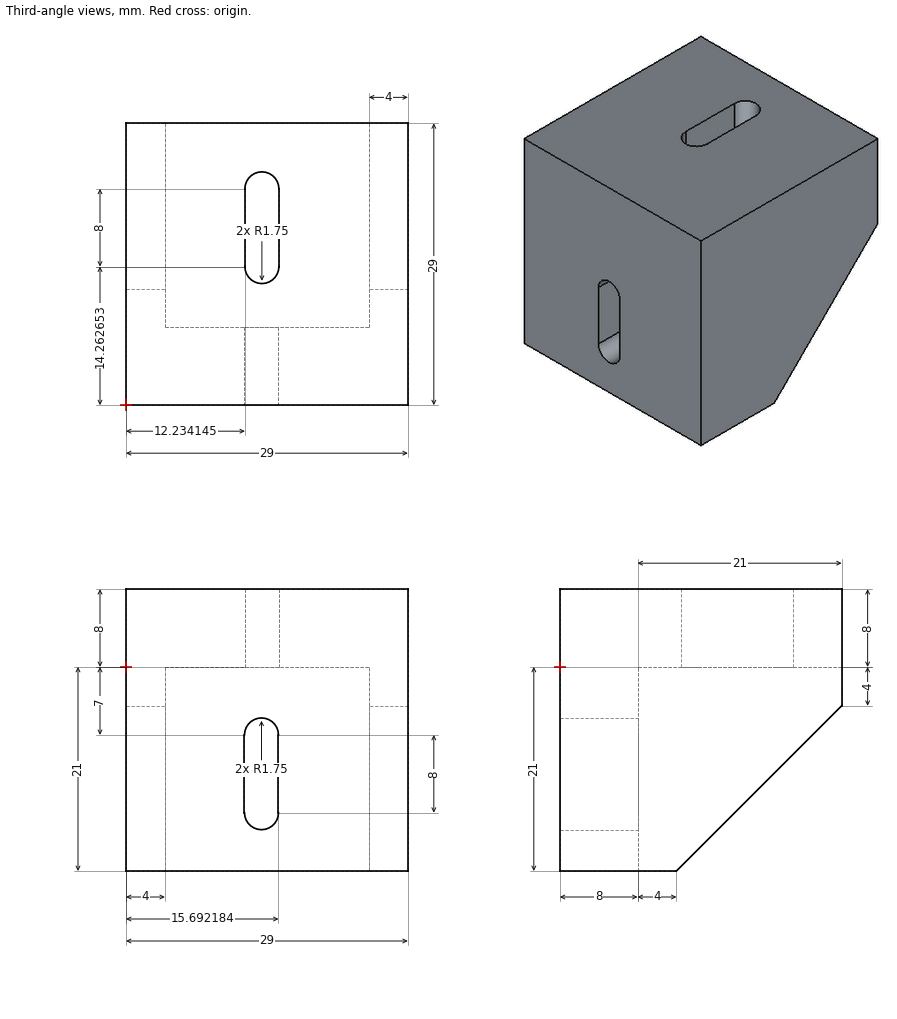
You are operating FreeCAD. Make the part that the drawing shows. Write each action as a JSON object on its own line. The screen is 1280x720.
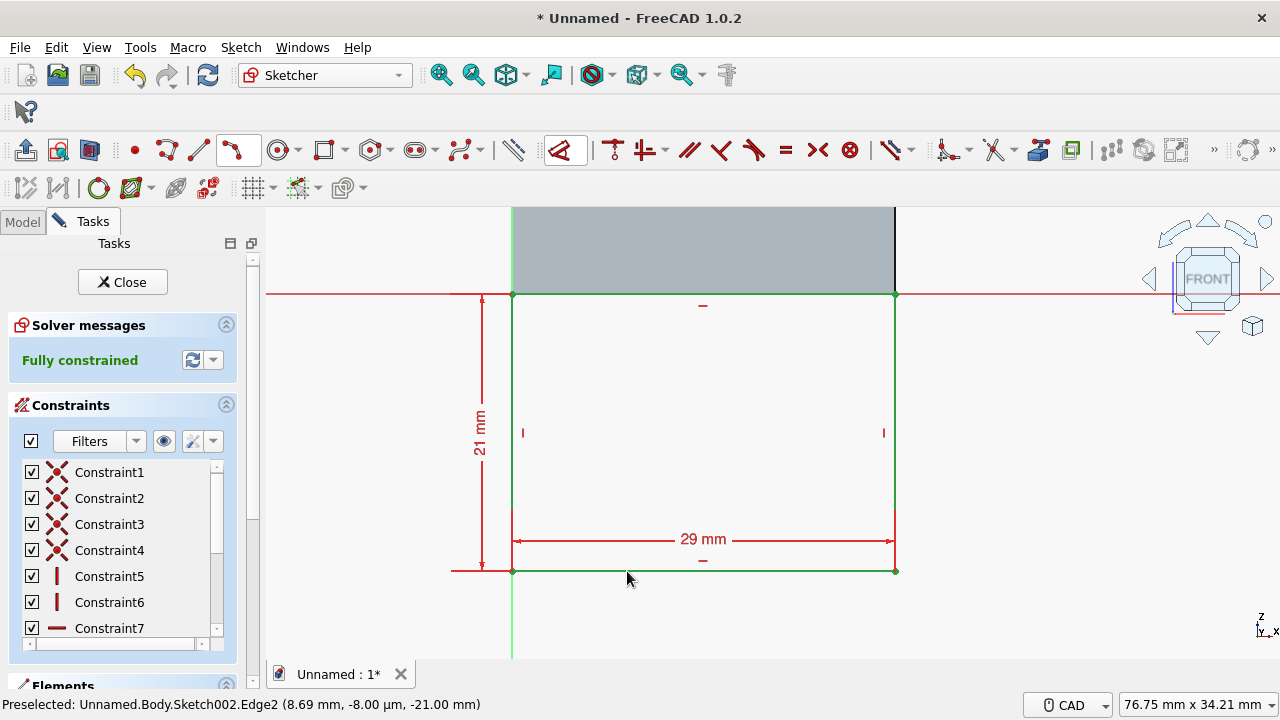
{"action": "left_click", "coordinate": [123, 282]}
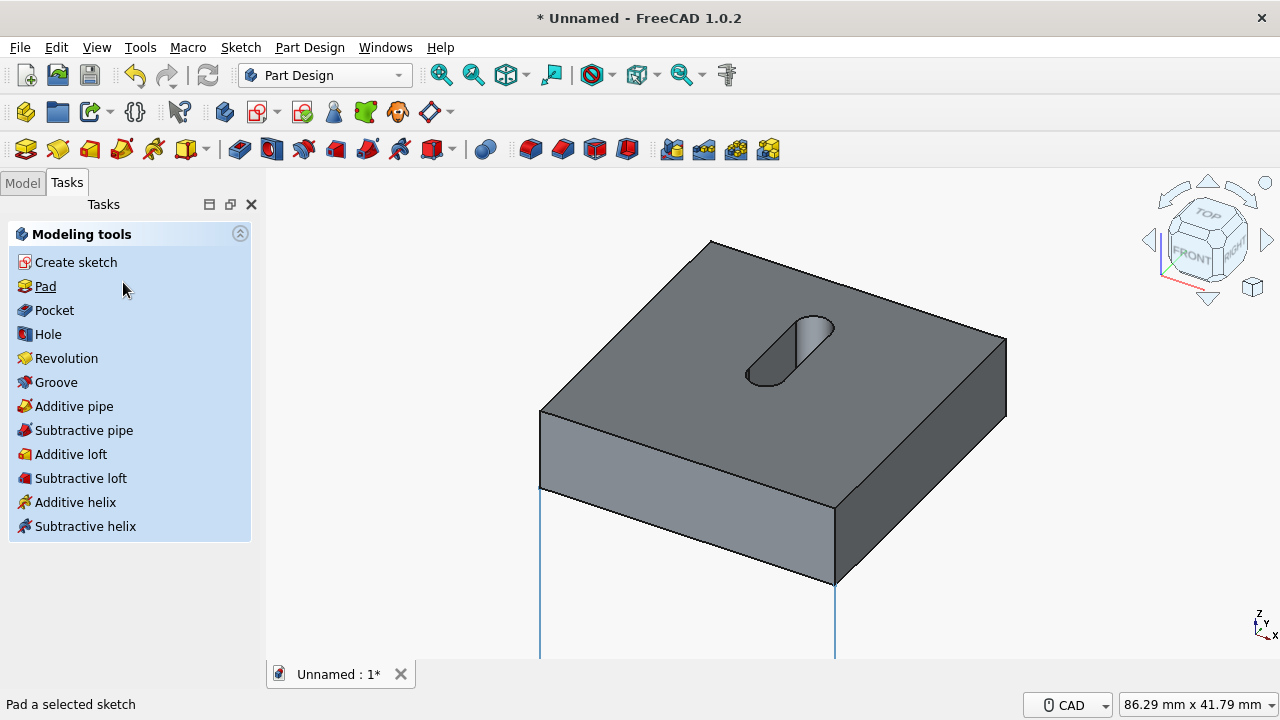
{"action": "left_click", "coordinate": [26, 150]}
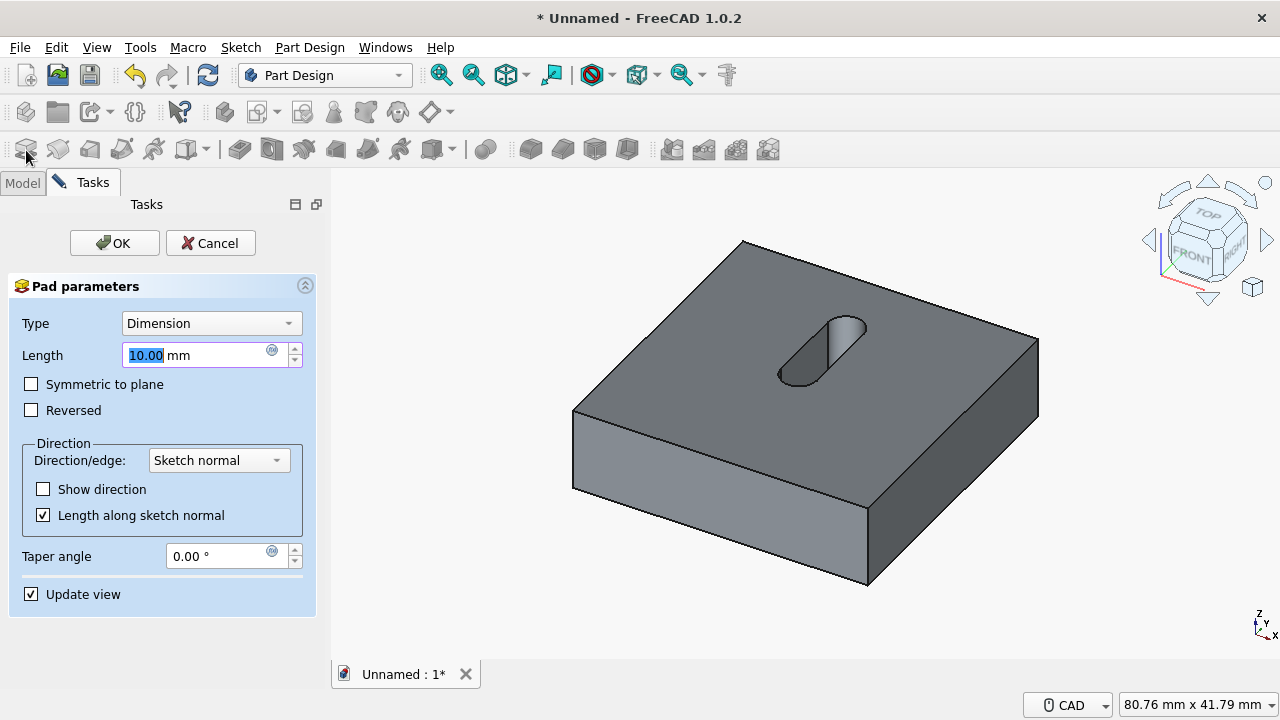
{"action": "type", "text": "8"}
{"action": "key", "text": "Tab"}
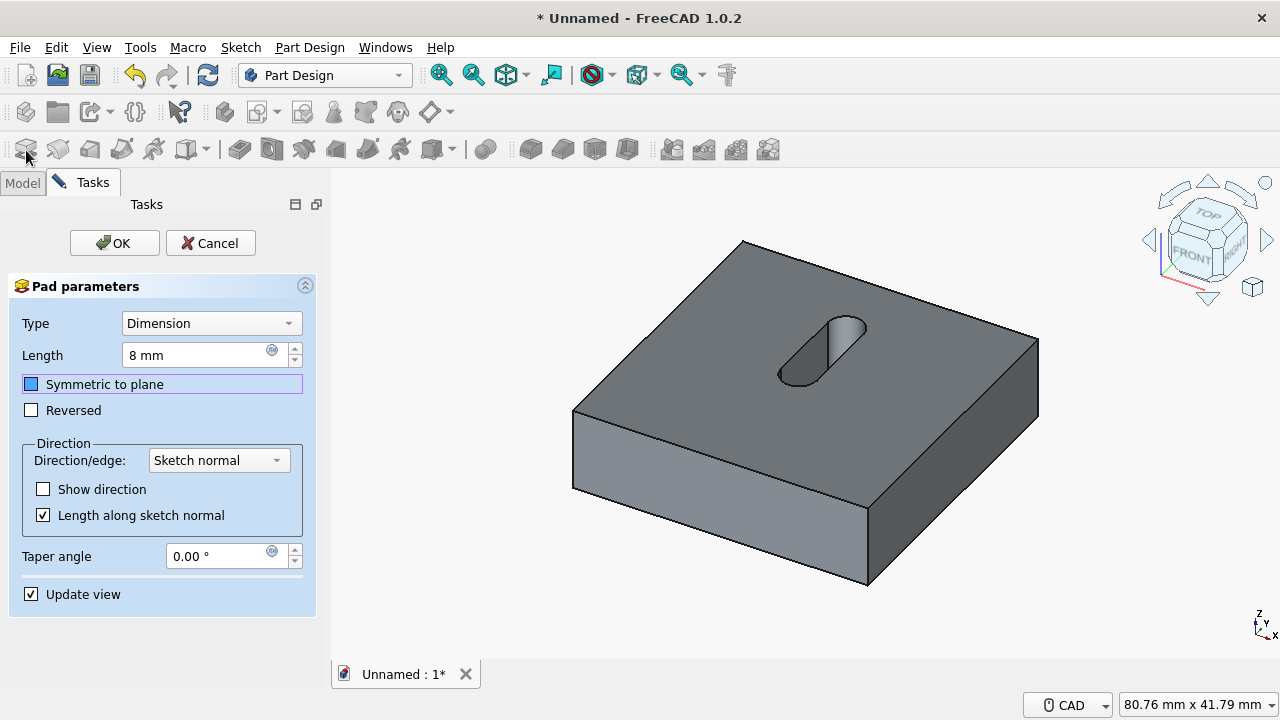
{"action": "left_click", "coordinate": [30, 410]}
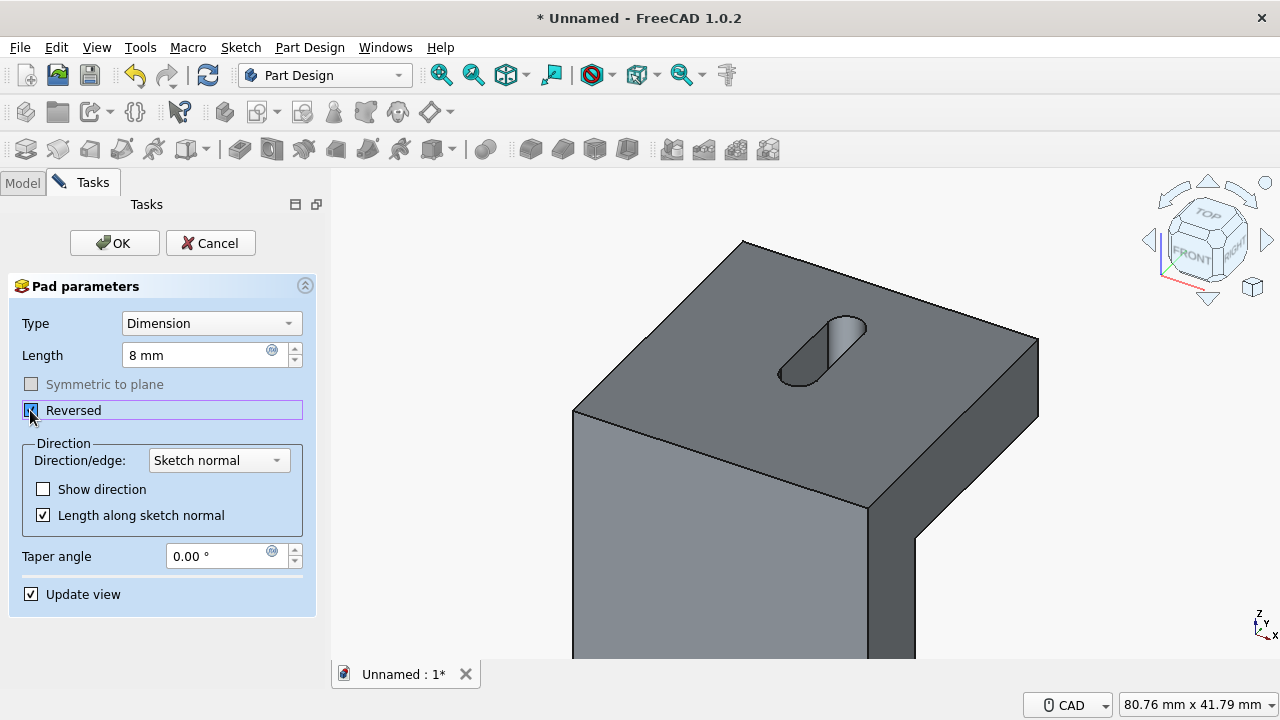
{"action": "left_click", "coordinate": [115, 243]}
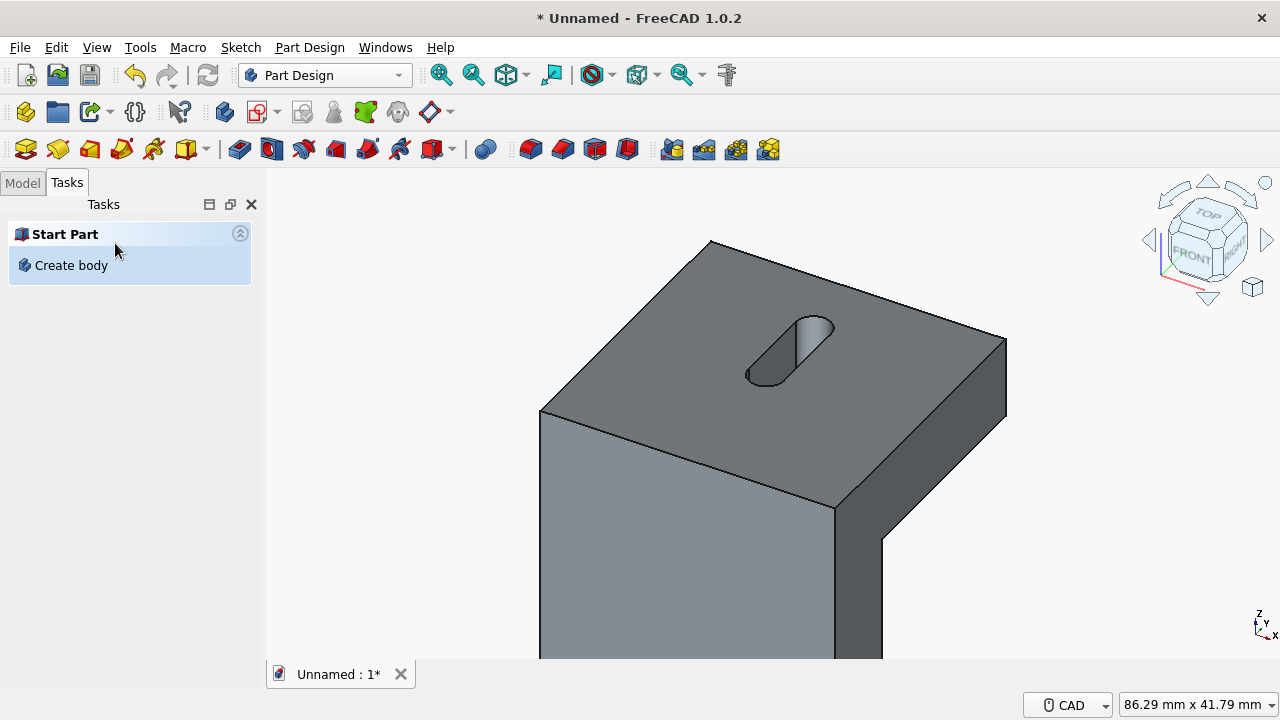
{"action": "key", "text": "v f"}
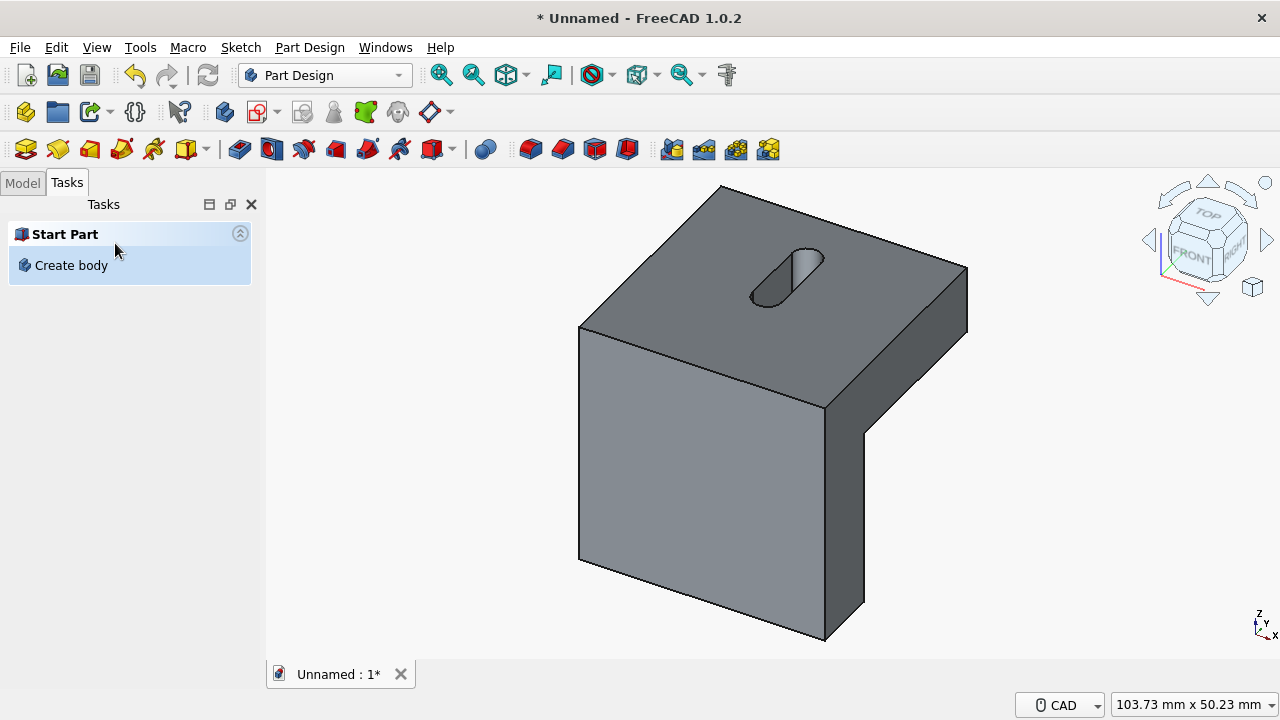
{"action": "key", "text": "4"}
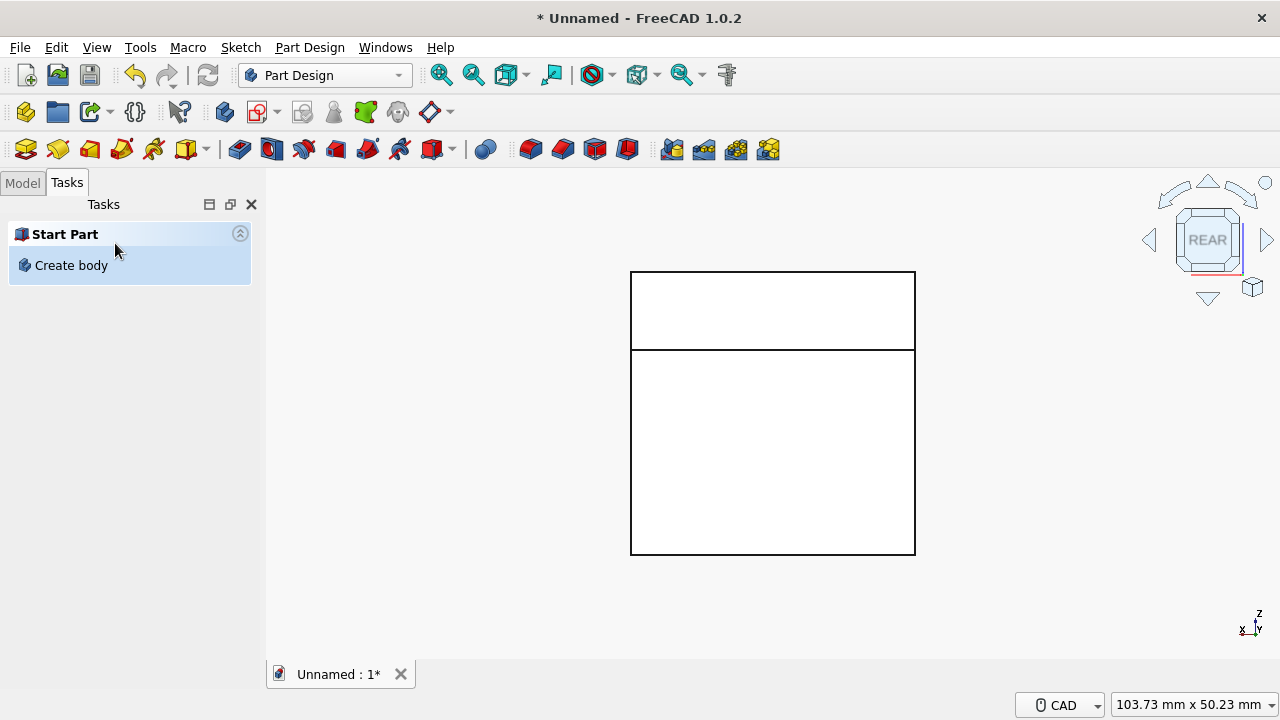
{"action": "left_click", "coordinate": [773, 452]}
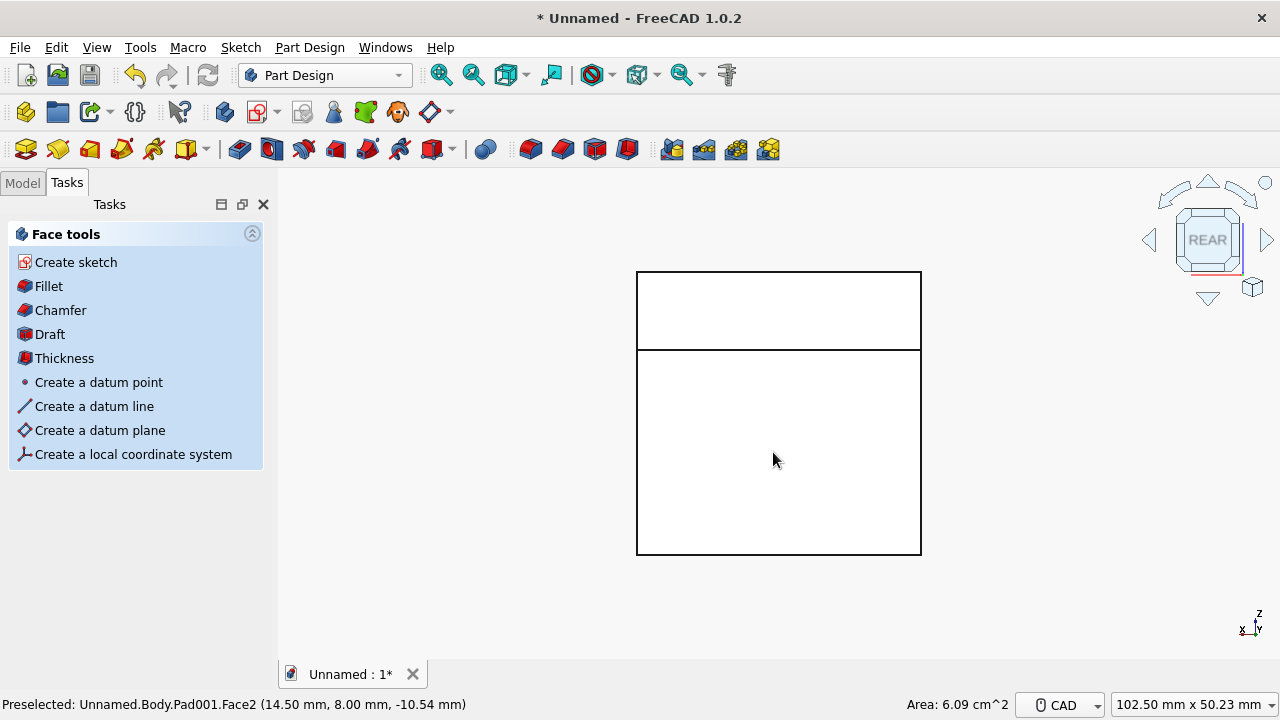
{"action": "left_click", "coordinate": [258, 112]}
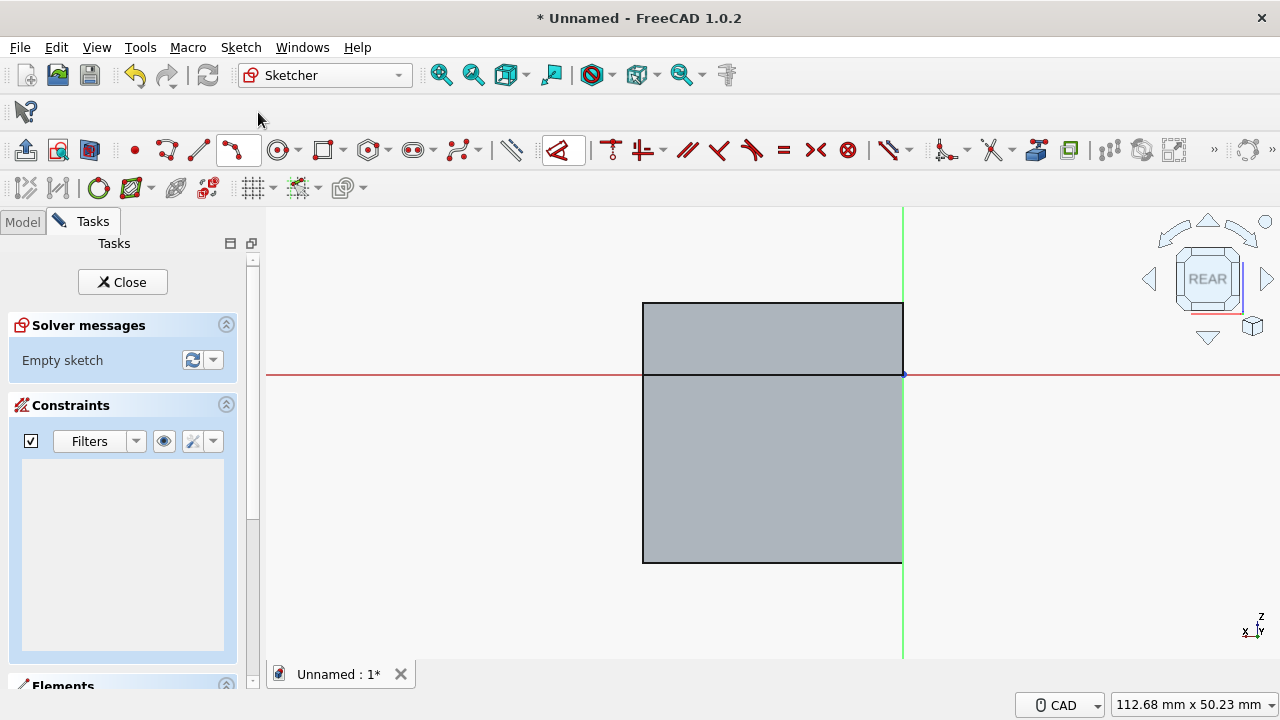
{"action": "left_click", "coordinate": [90, 150]}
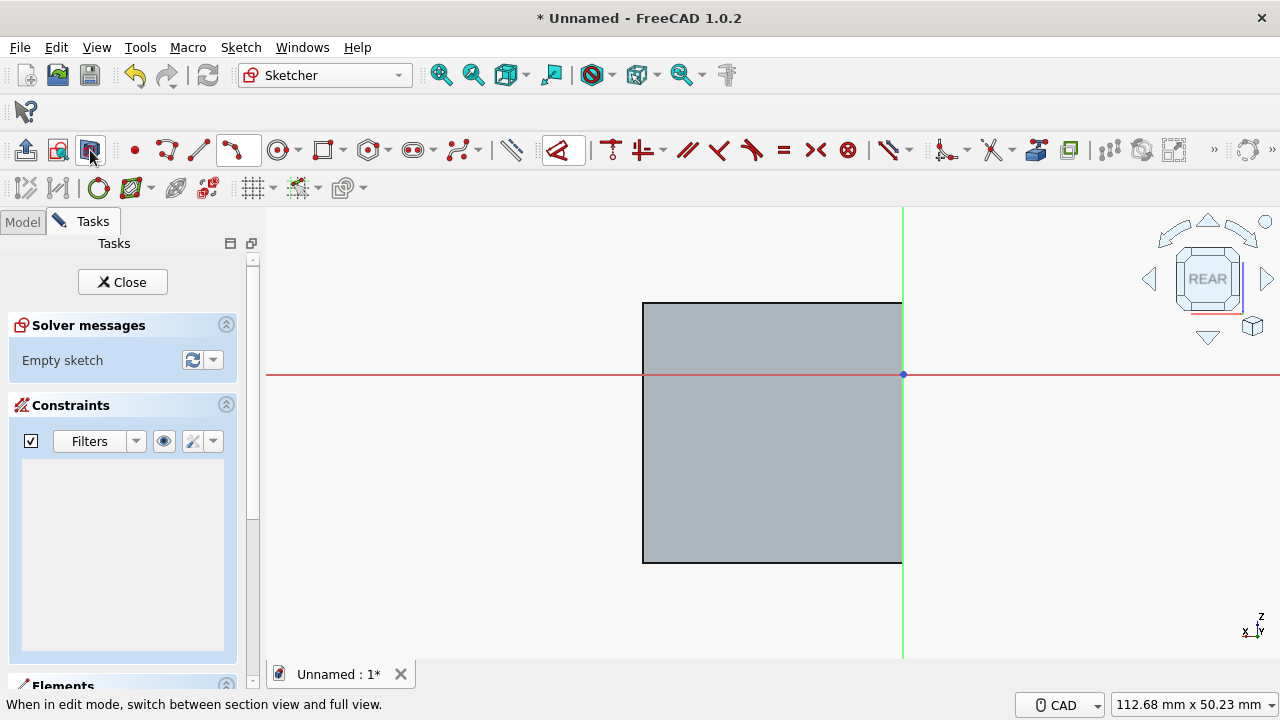
{"action": "scroll", "coordinate": [989, 470], "scroll_direction": "up", "scroll_amount": 3}